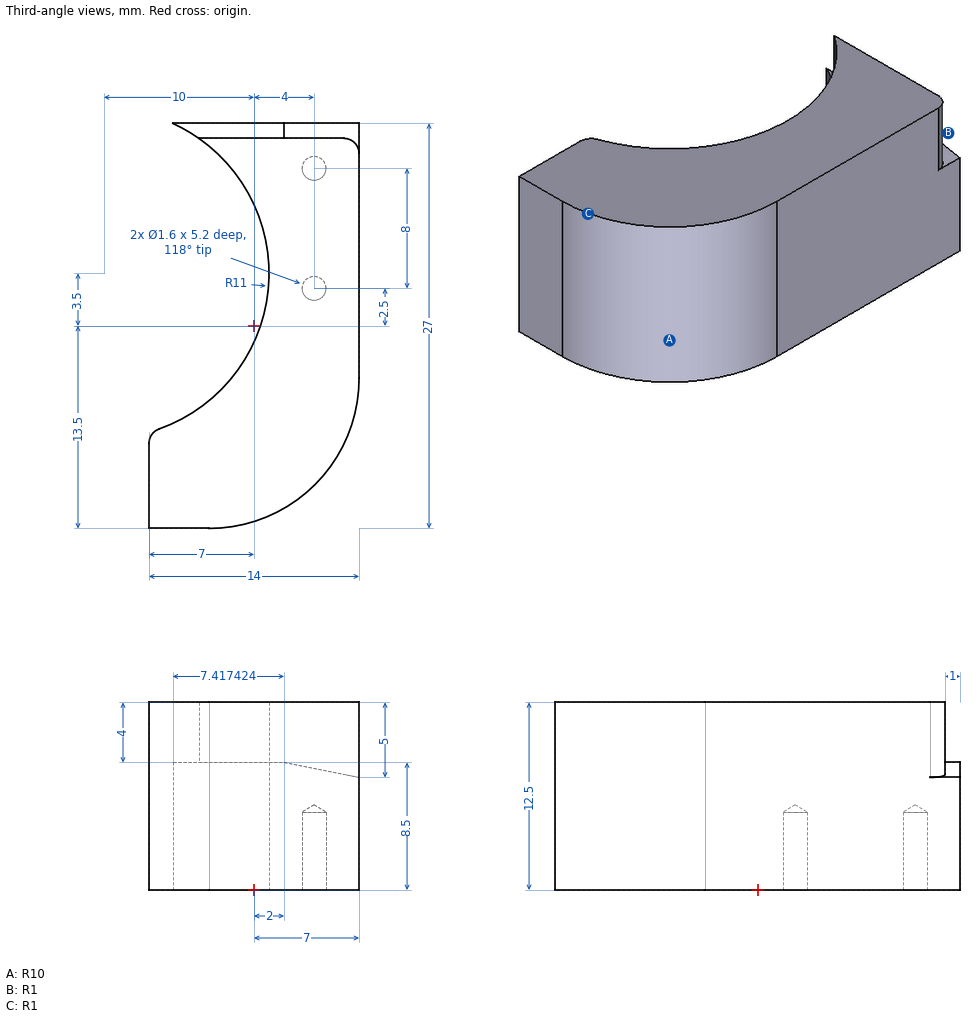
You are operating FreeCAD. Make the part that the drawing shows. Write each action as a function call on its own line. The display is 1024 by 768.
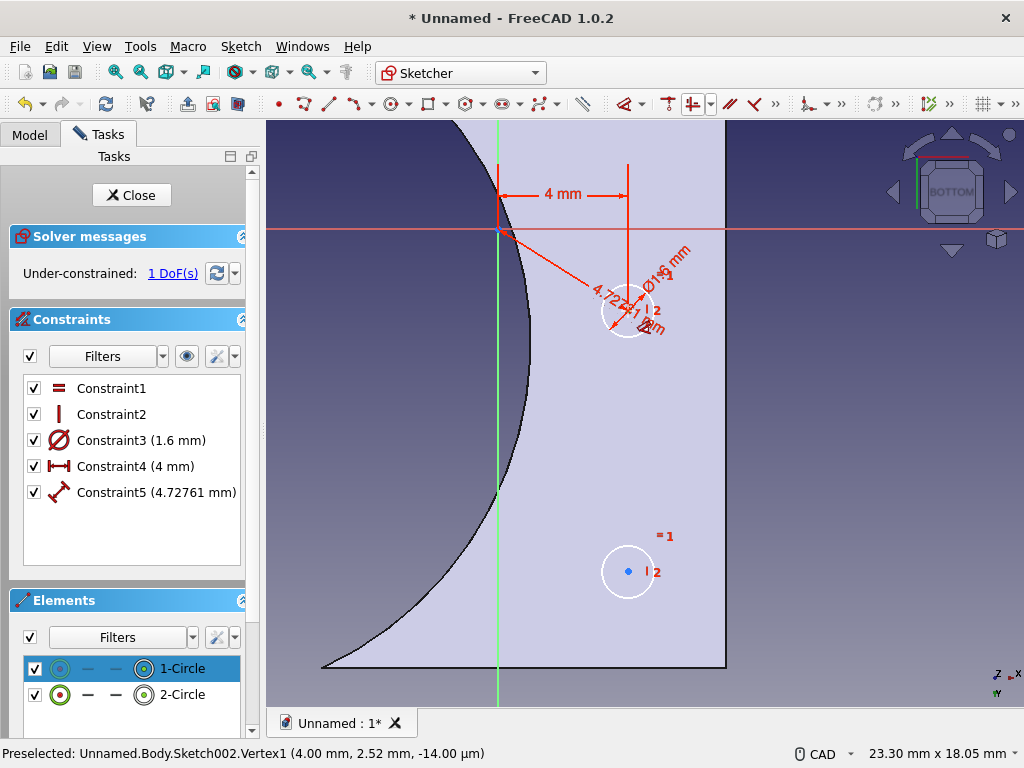
click(628, 572)
click(662, 442)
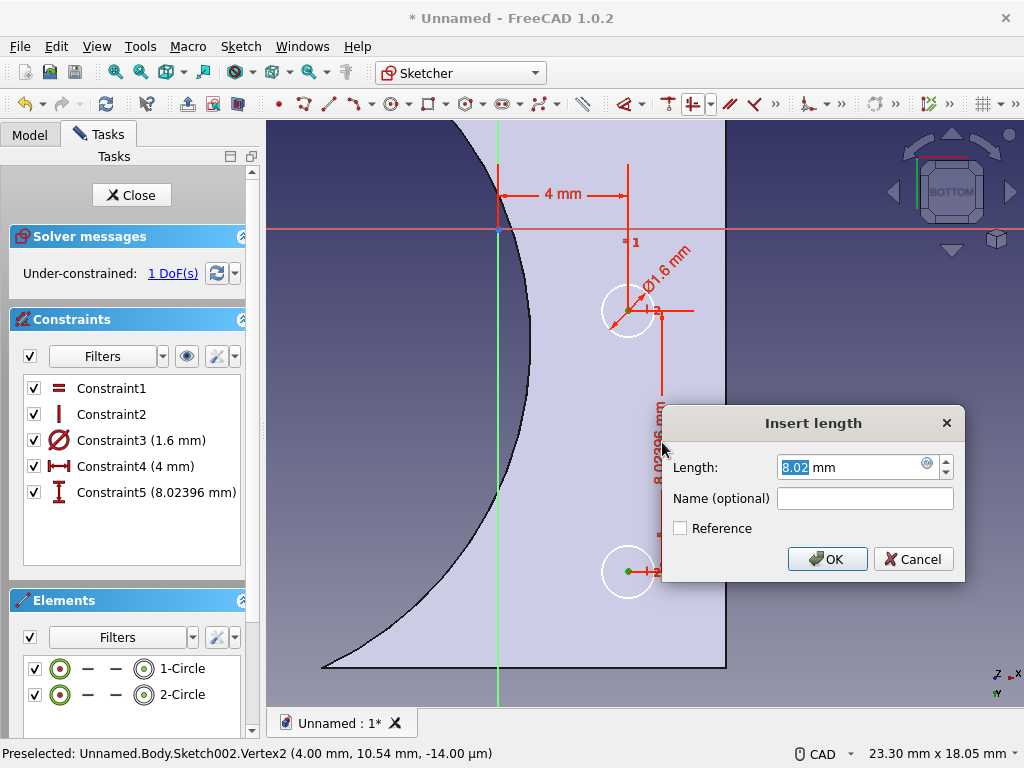
text(8)
key(Return)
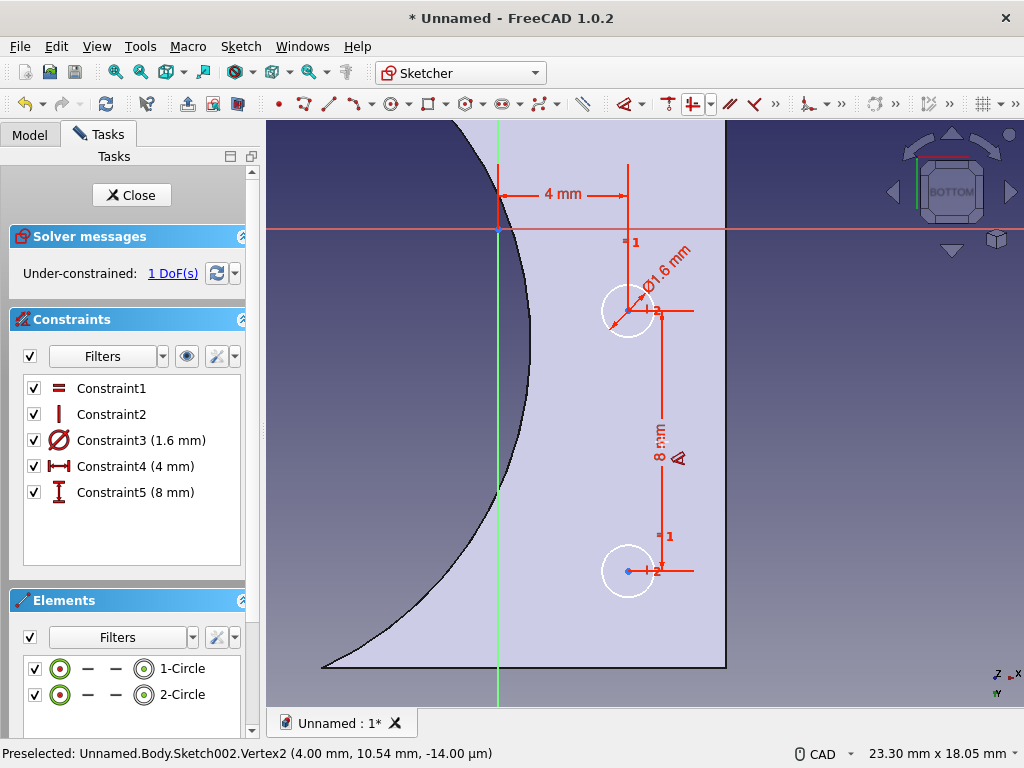
click(628, 311)
click(464, 270)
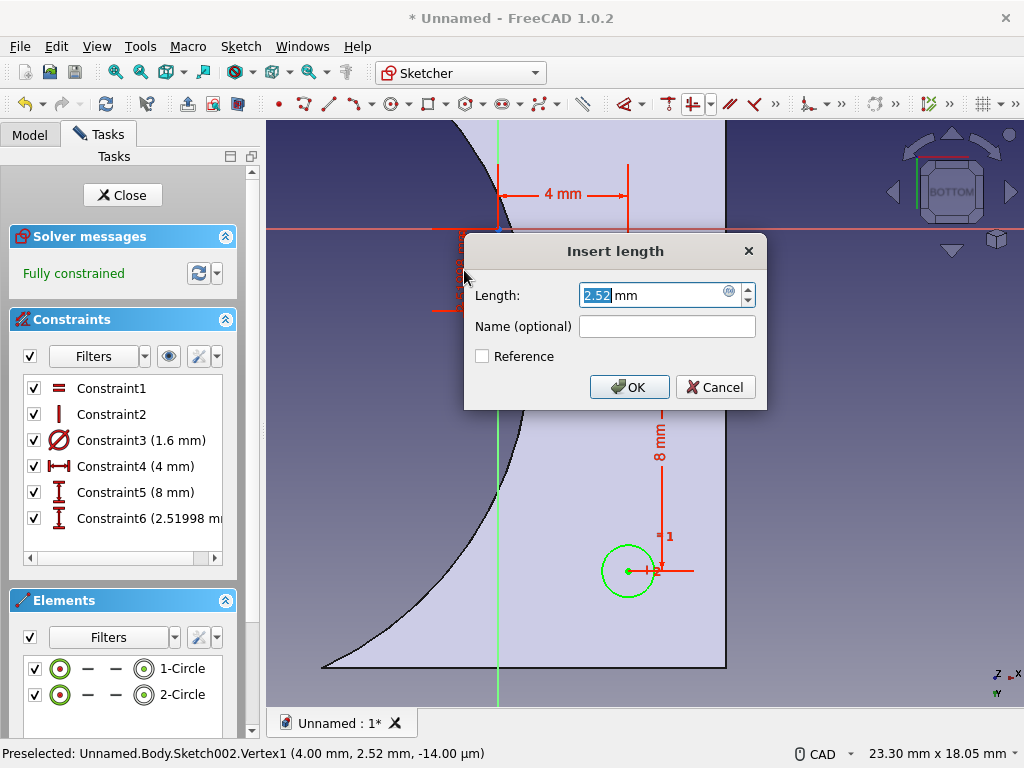
text(2.5)
key(Return)
key(Escape)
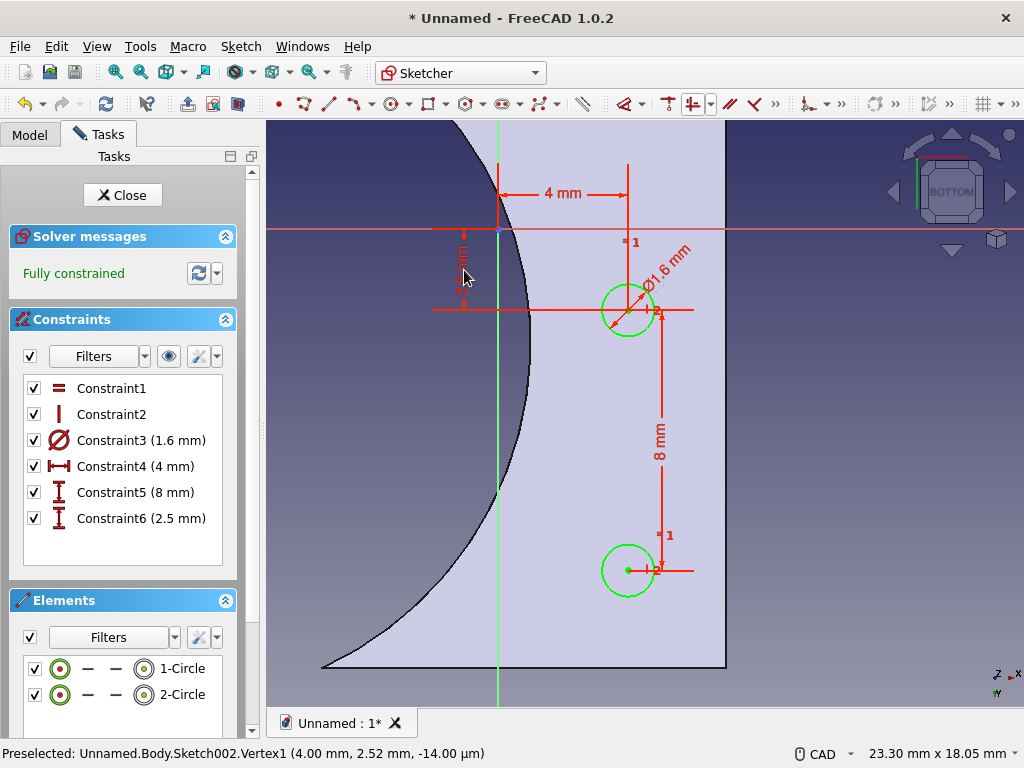
click(123, 195)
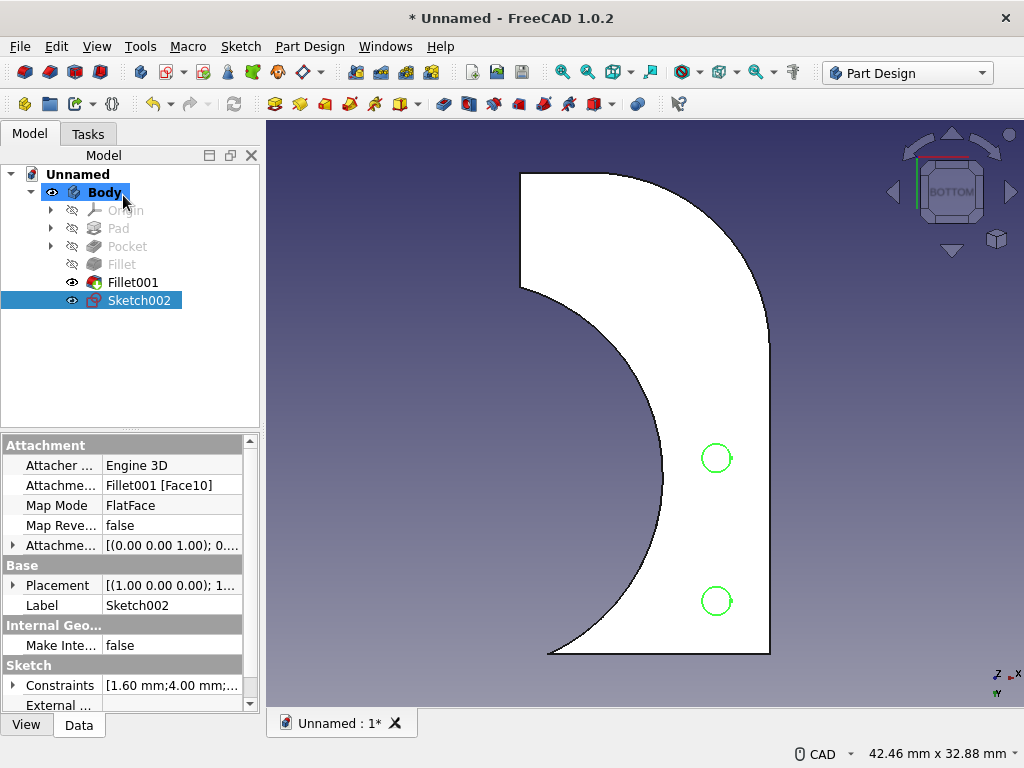
click(469, 104)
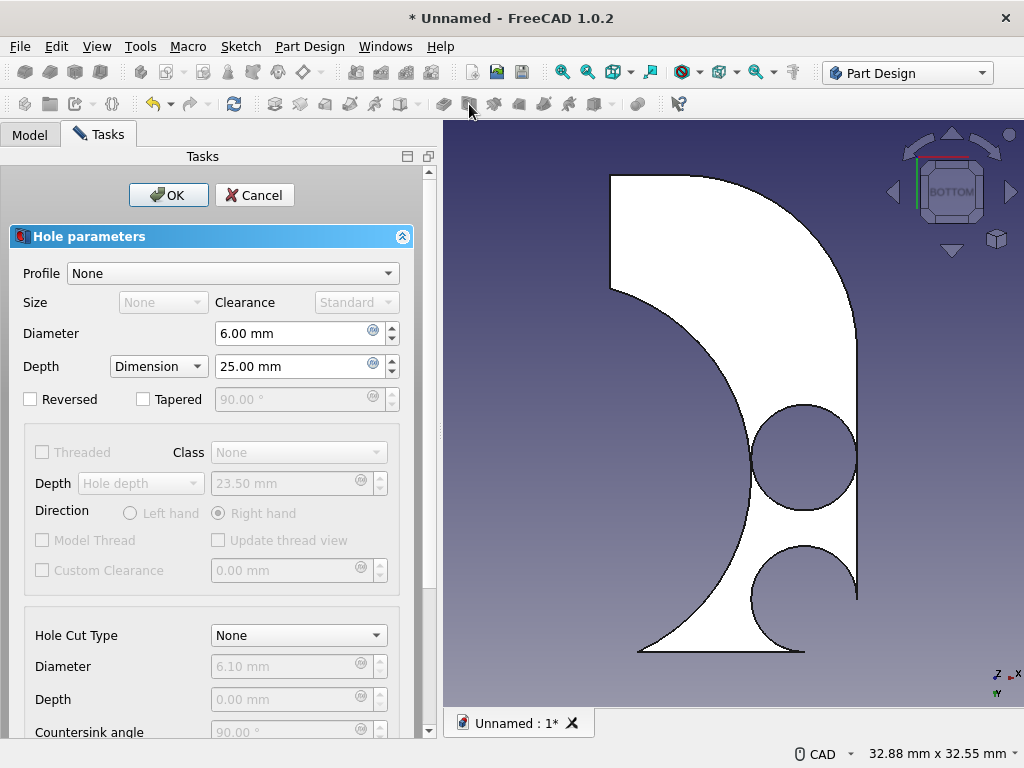
triple_click(300, 334)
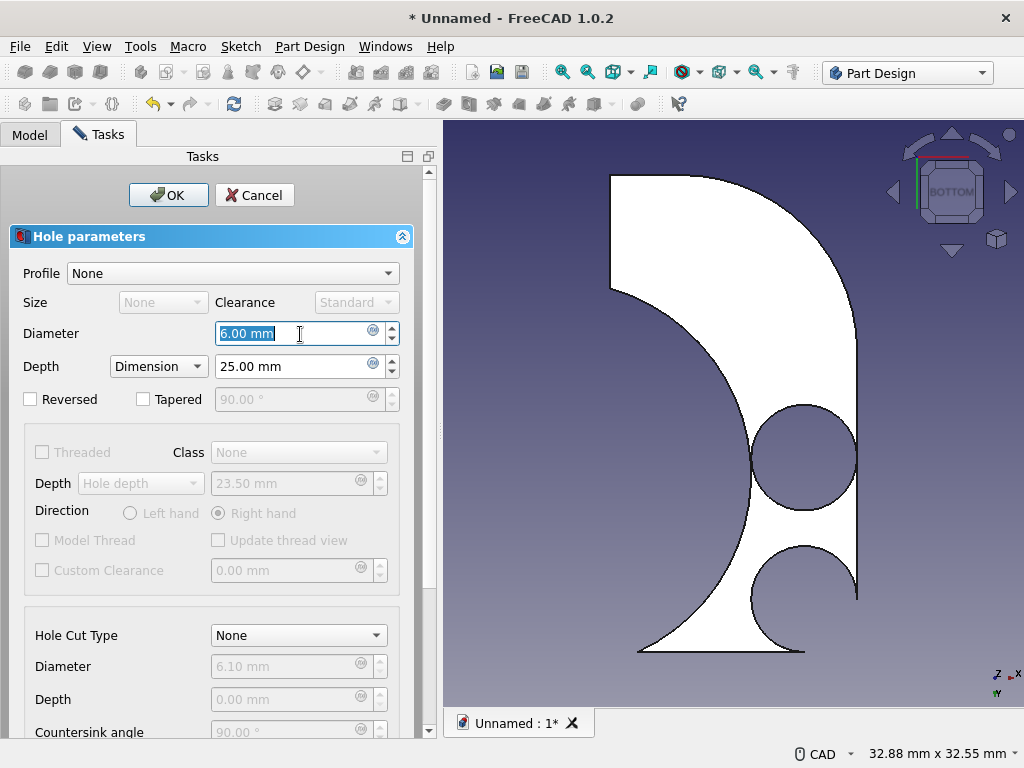
text(1.6)
key(Tab)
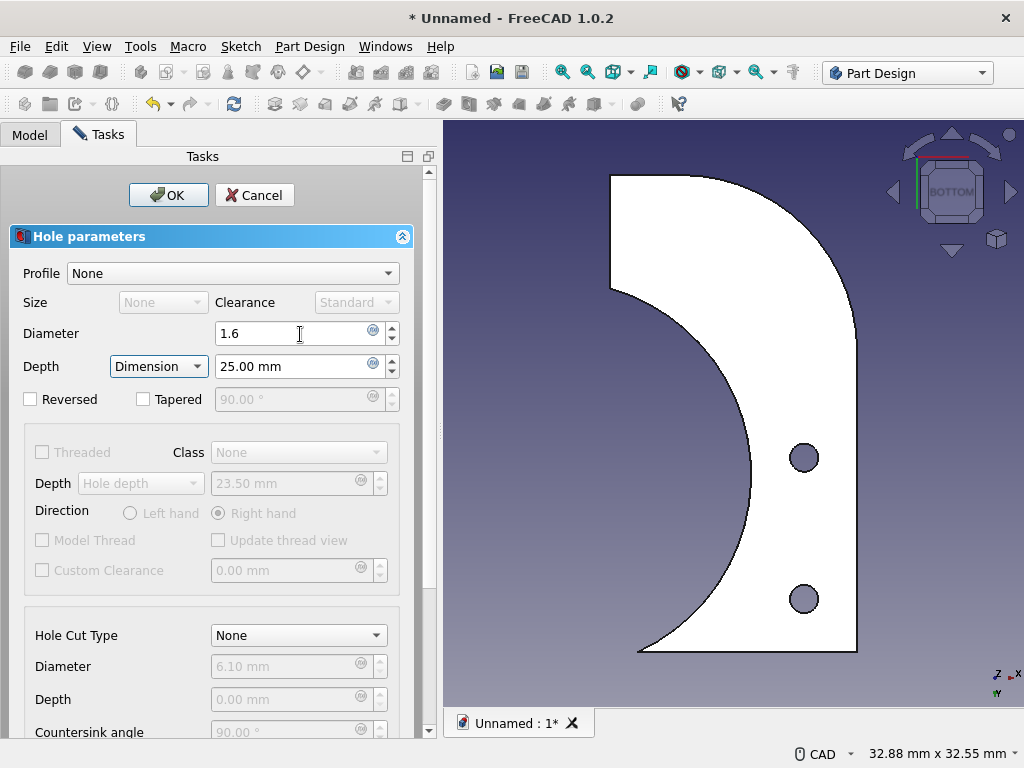
triple_click(300, 366)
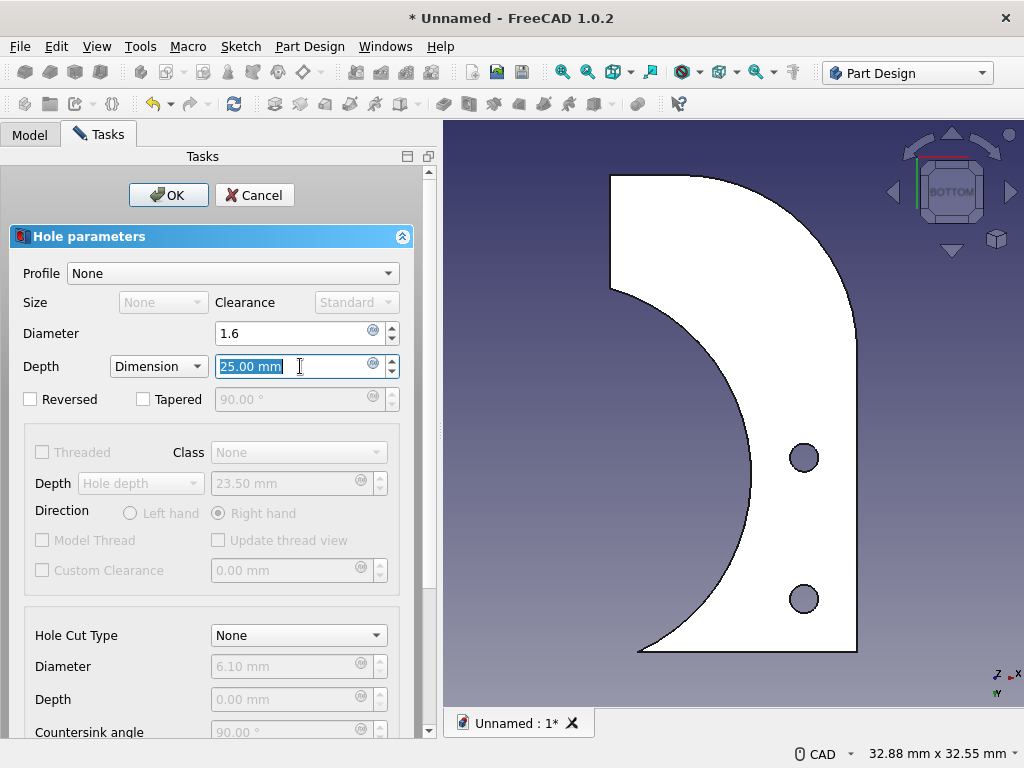
text(5.2)
key(Tab)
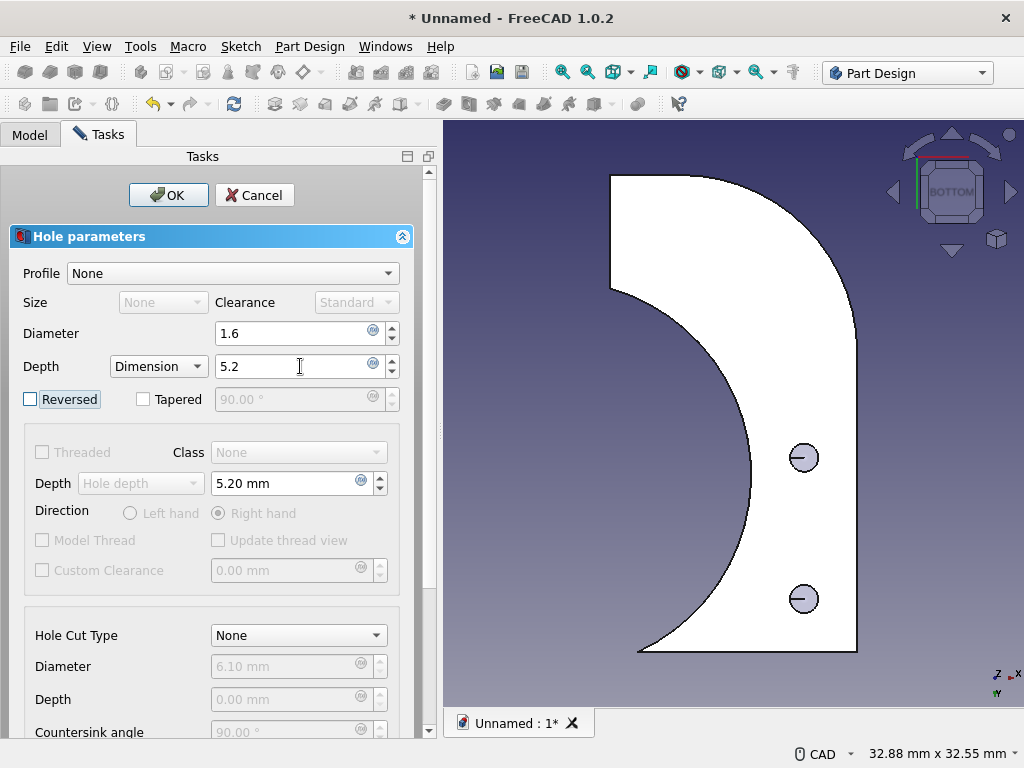
click(169, 195)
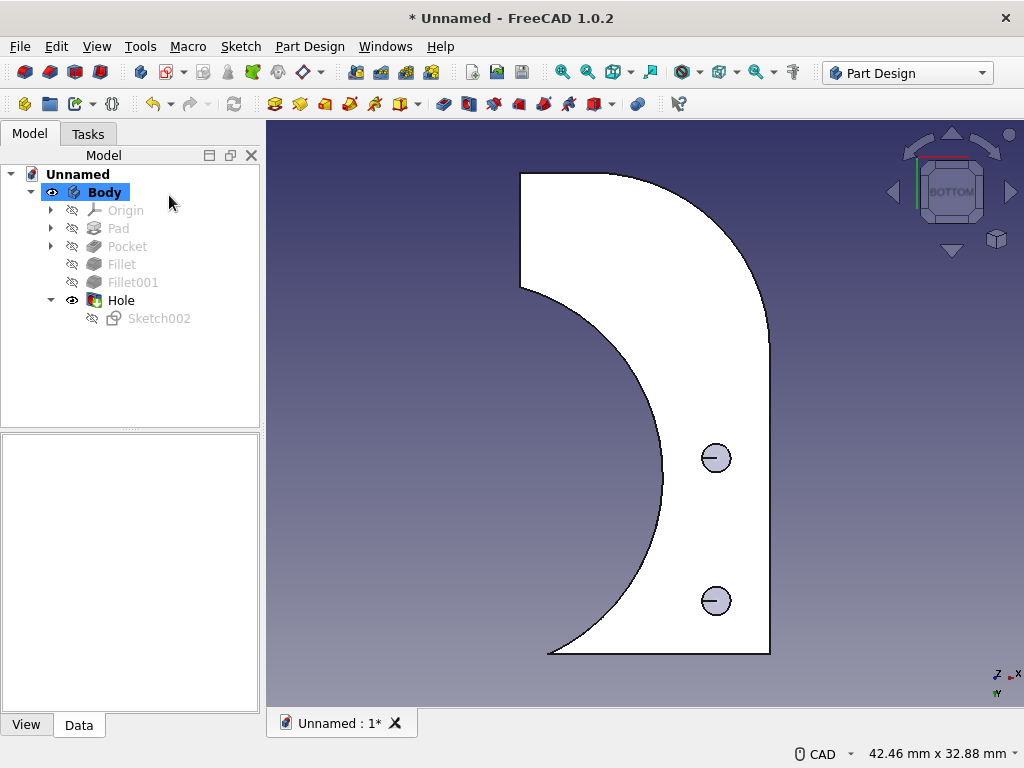
key(0)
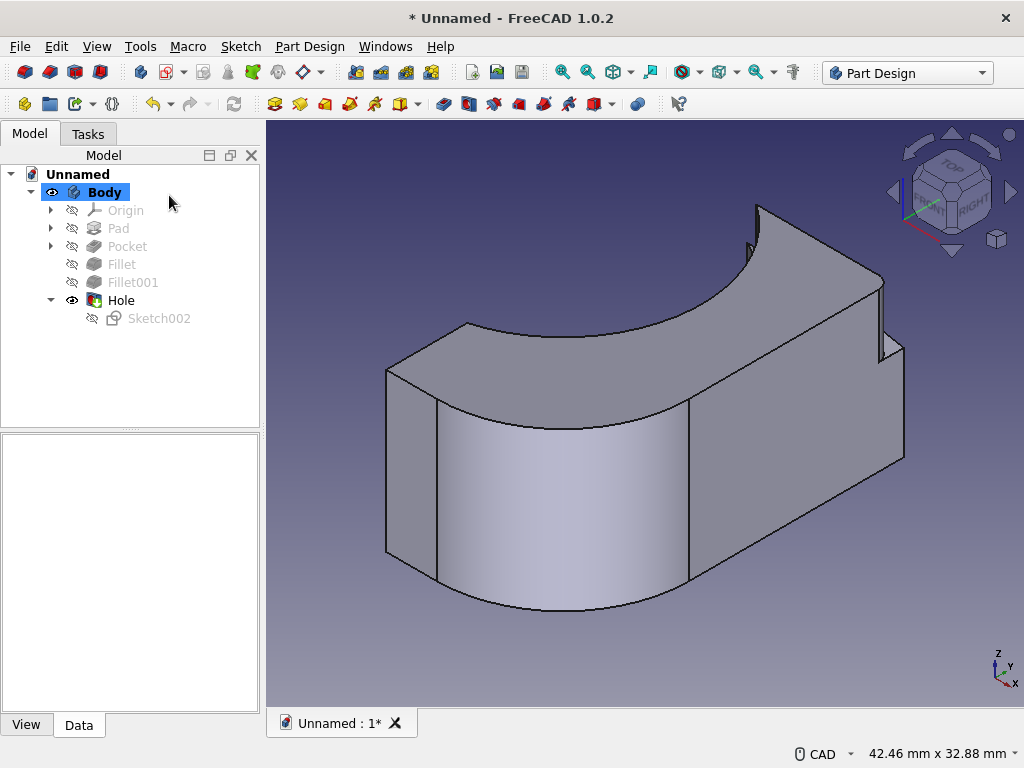
key(2)